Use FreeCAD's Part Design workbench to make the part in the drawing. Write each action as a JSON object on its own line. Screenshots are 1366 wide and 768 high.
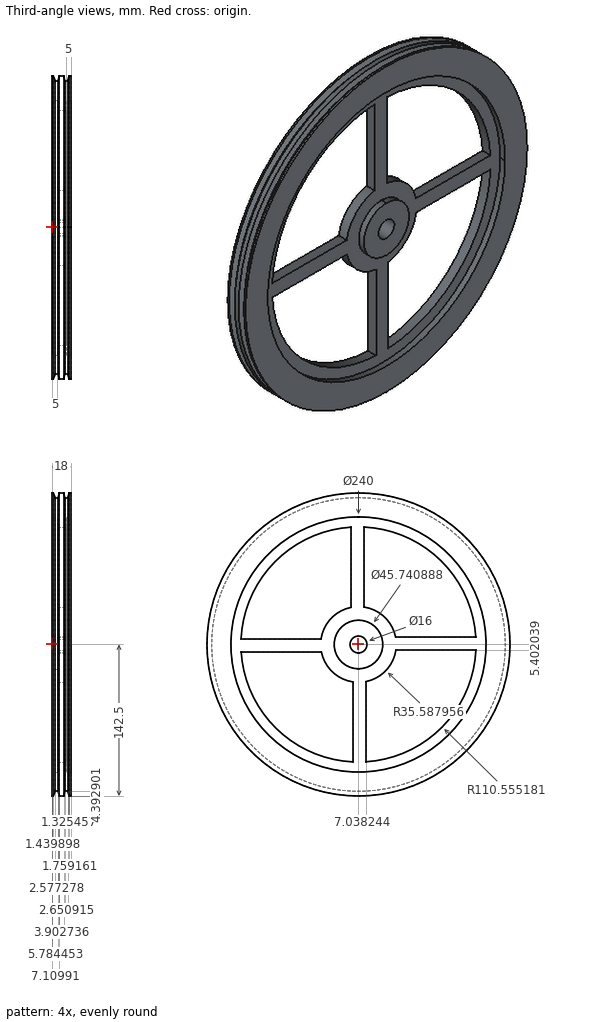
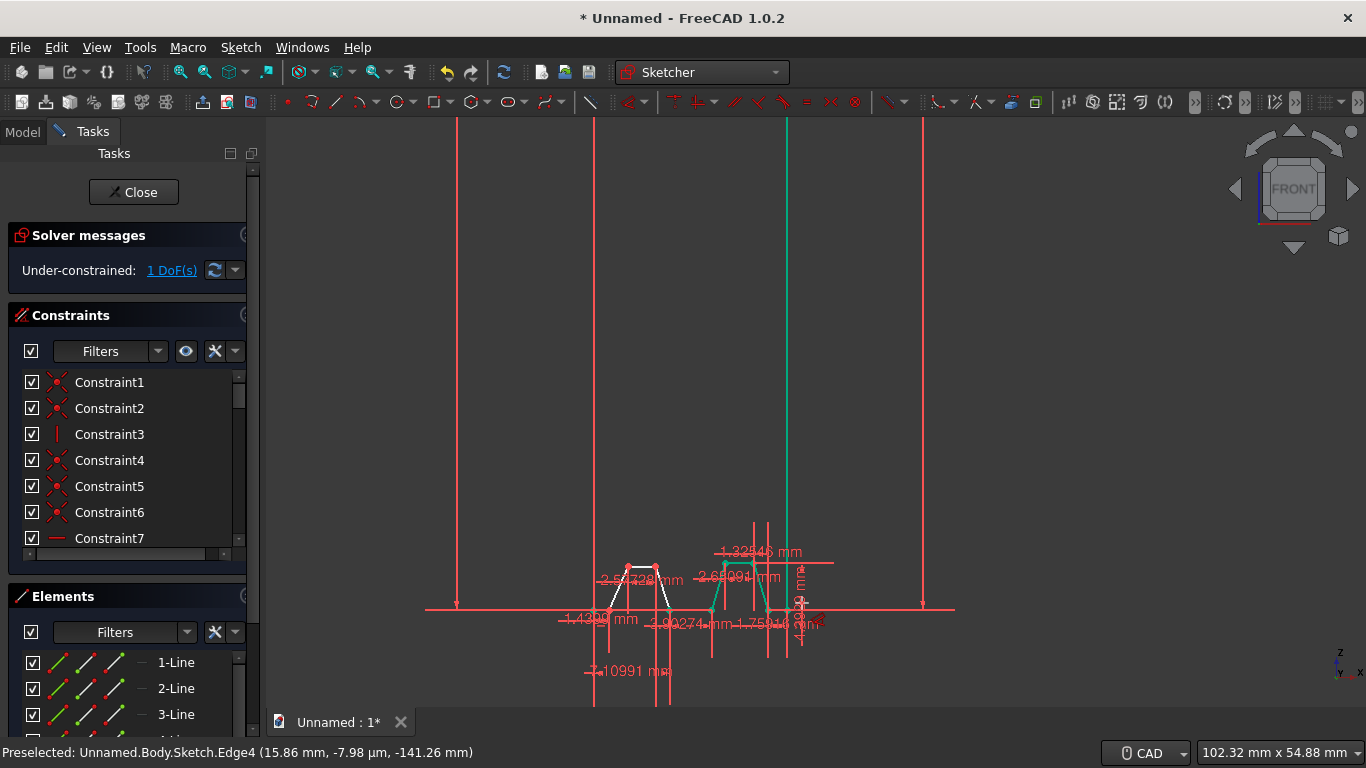
{"action": "left_click", "coordinate": [666, 597]}
{"action": "left_click", "coordinate": [728, 604]}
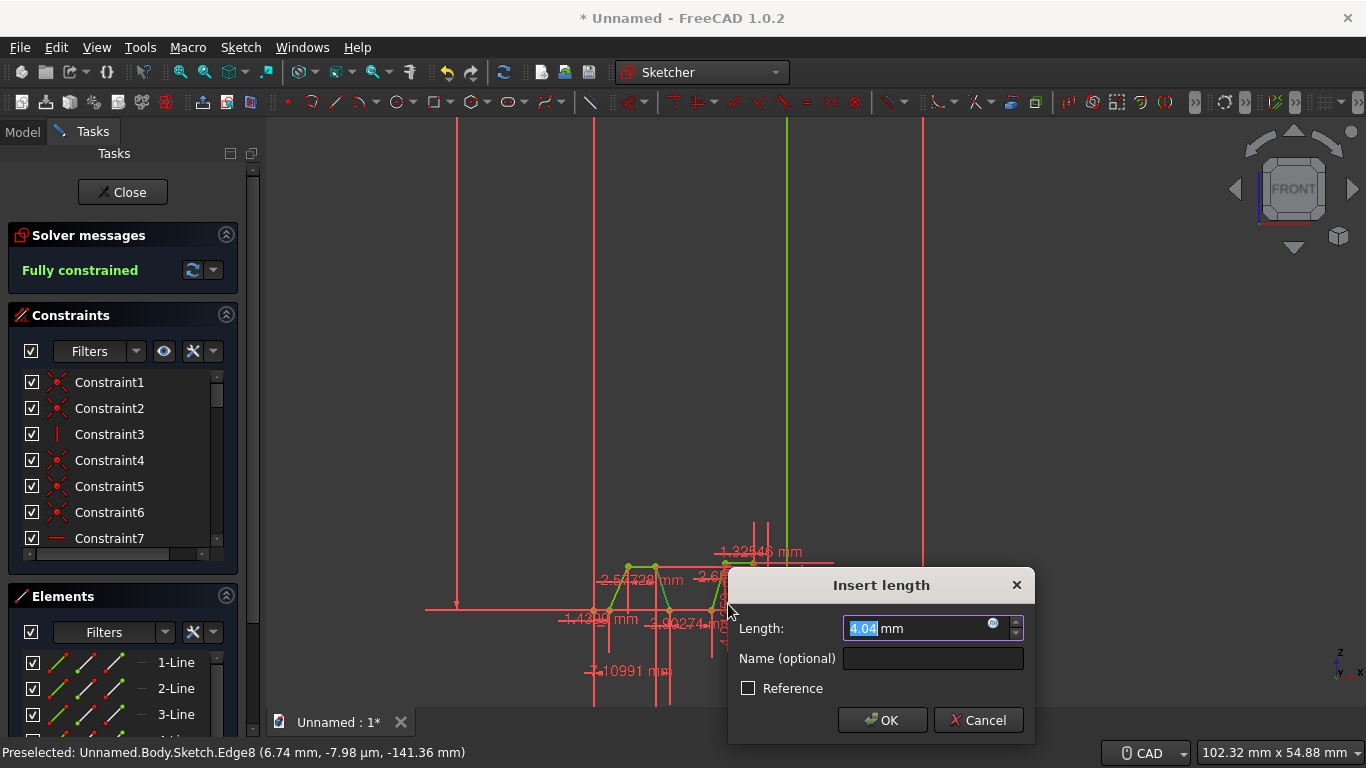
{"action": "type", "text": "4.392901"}
{"action": "key", "text": "Return"}
{"action": "key", "text": "Escape"}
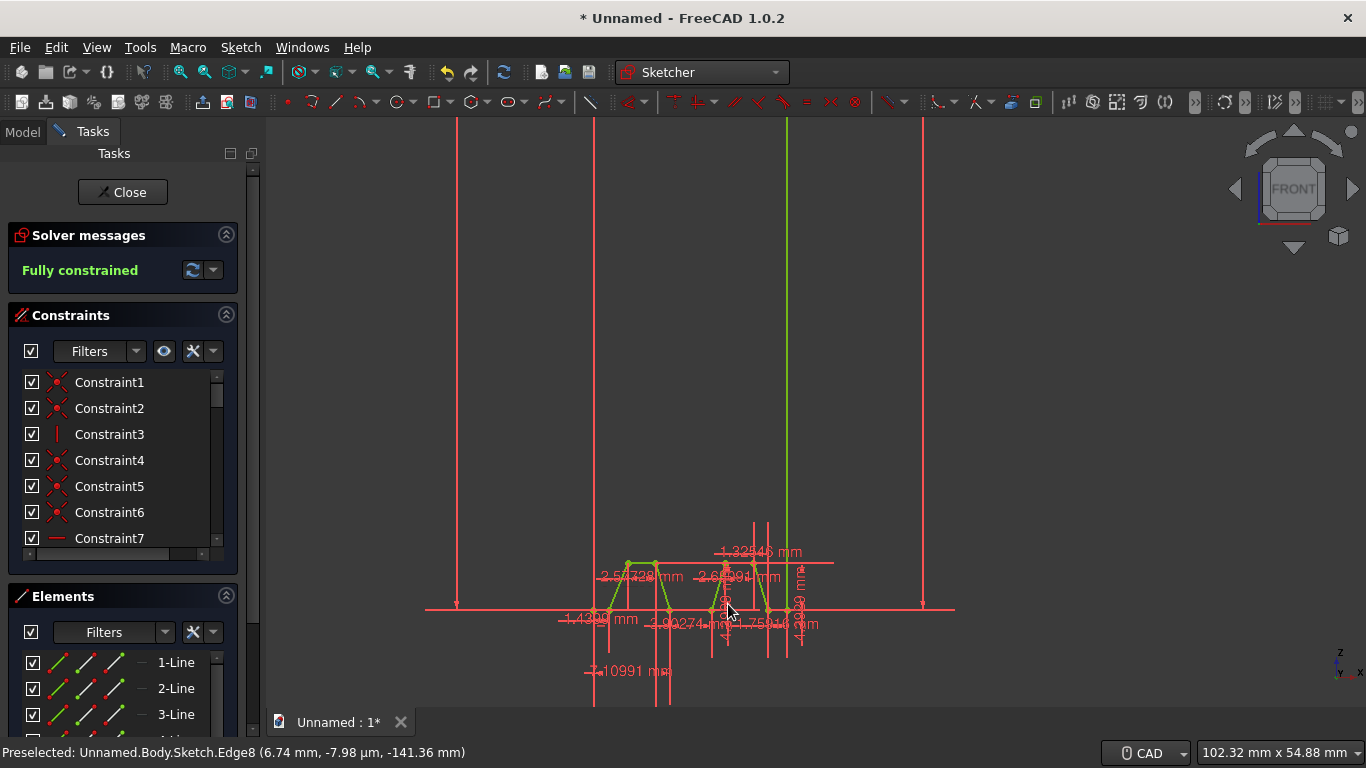
{"action": "left_click", "coordinate": [123, 192]}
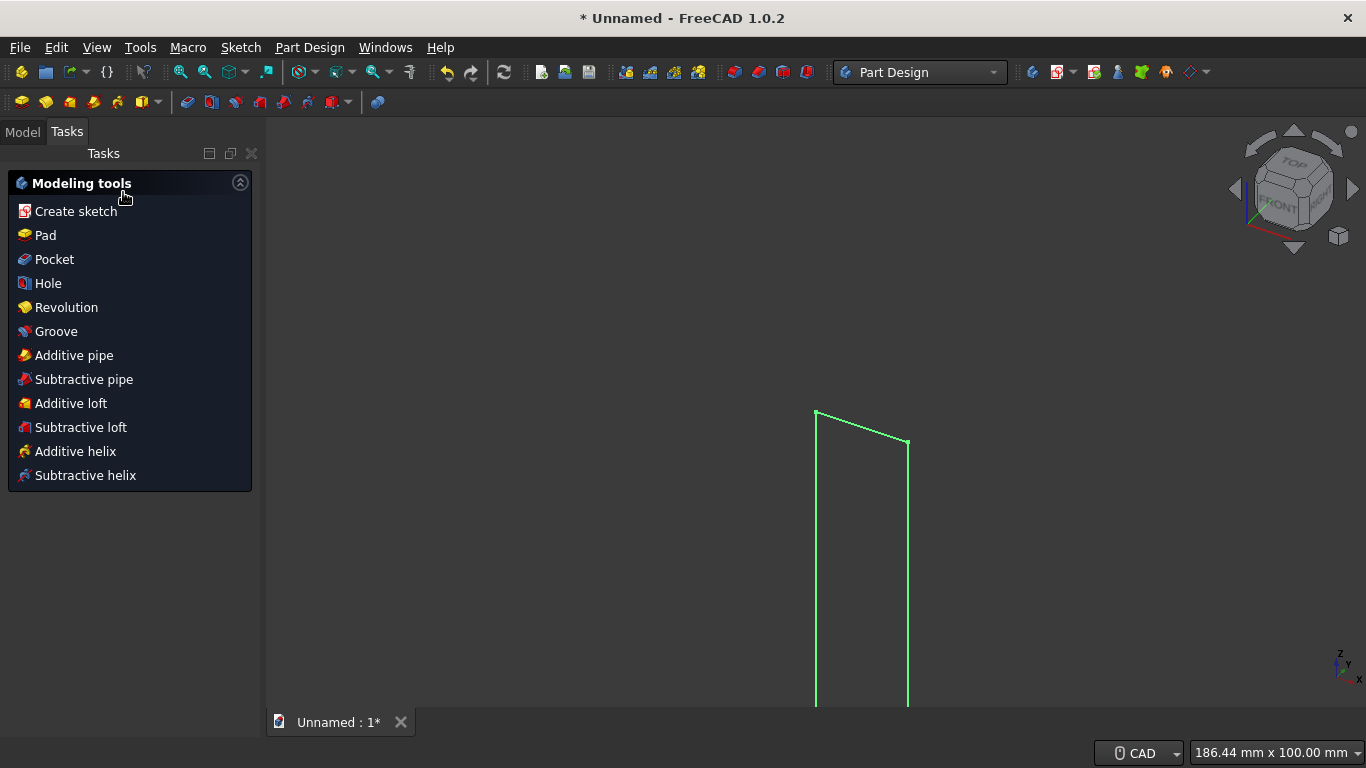
{"action": "left_click", "coordinate": [46, 102]}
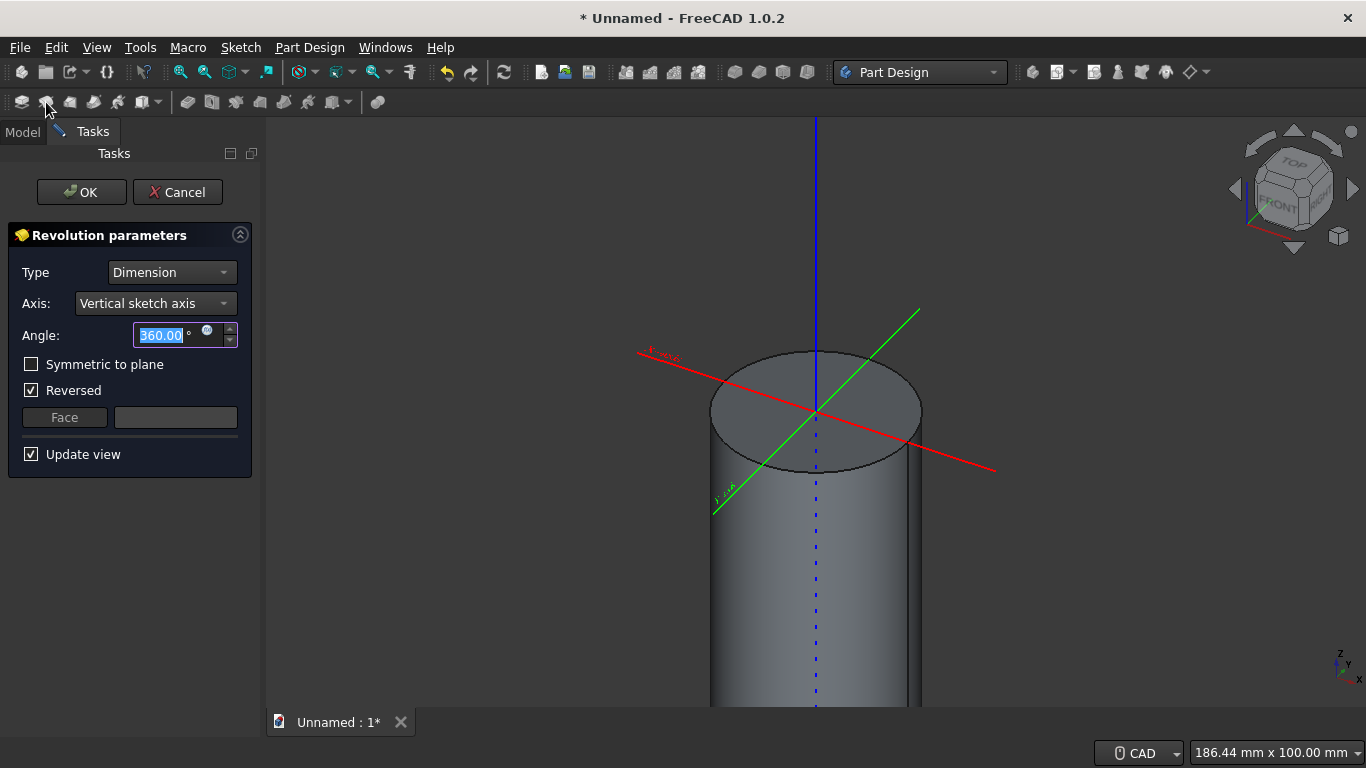
{"action": "left_click", "coordinate": [156, 304]}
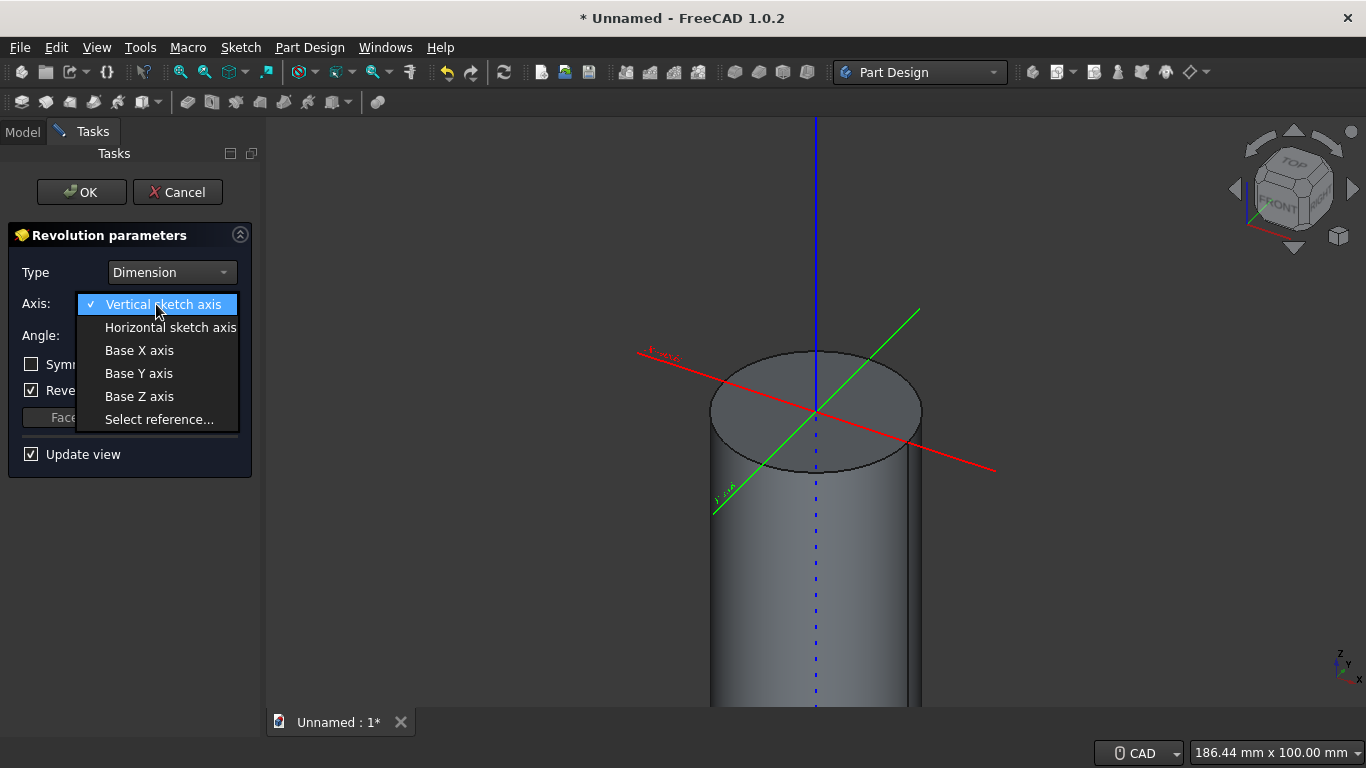
{"action": "left_click", "coordinate": [156, 328]}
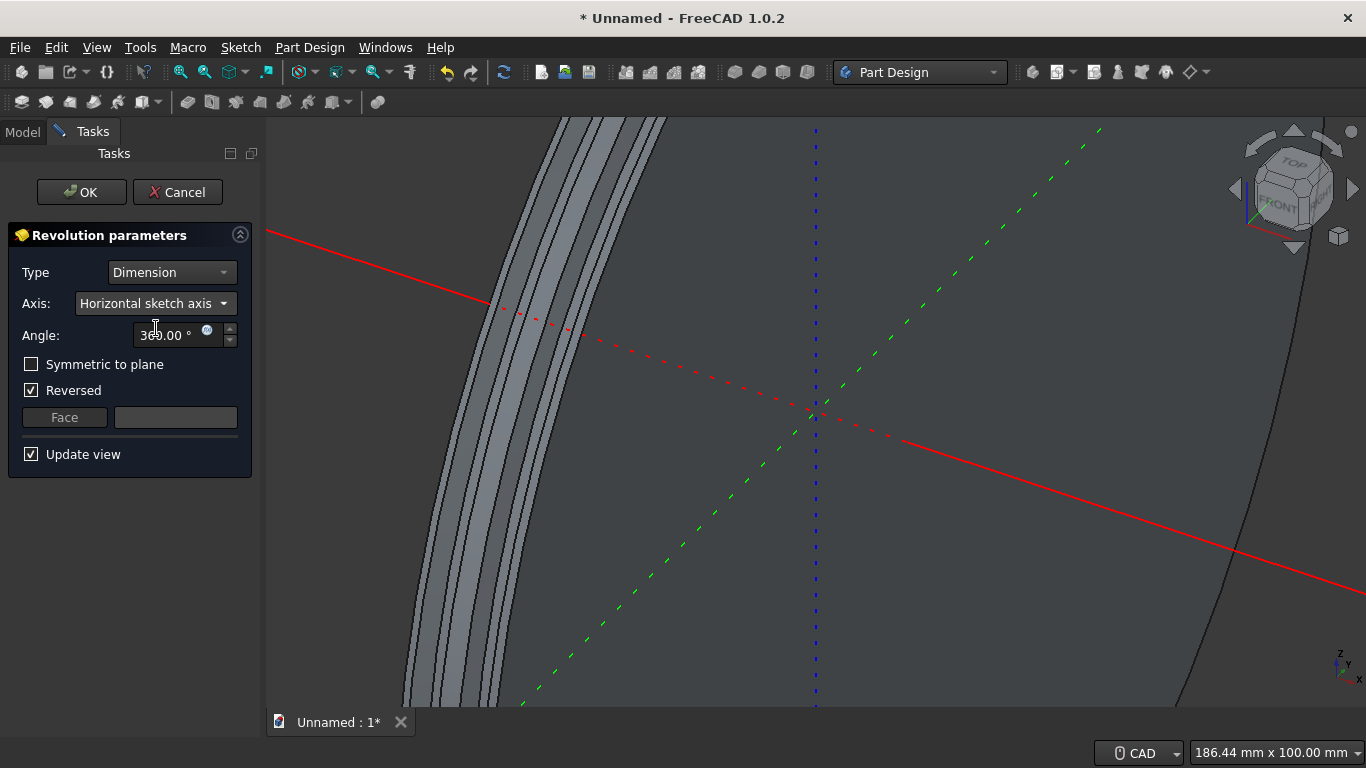
{"action": "left_click", "coordinate": [82, 192]}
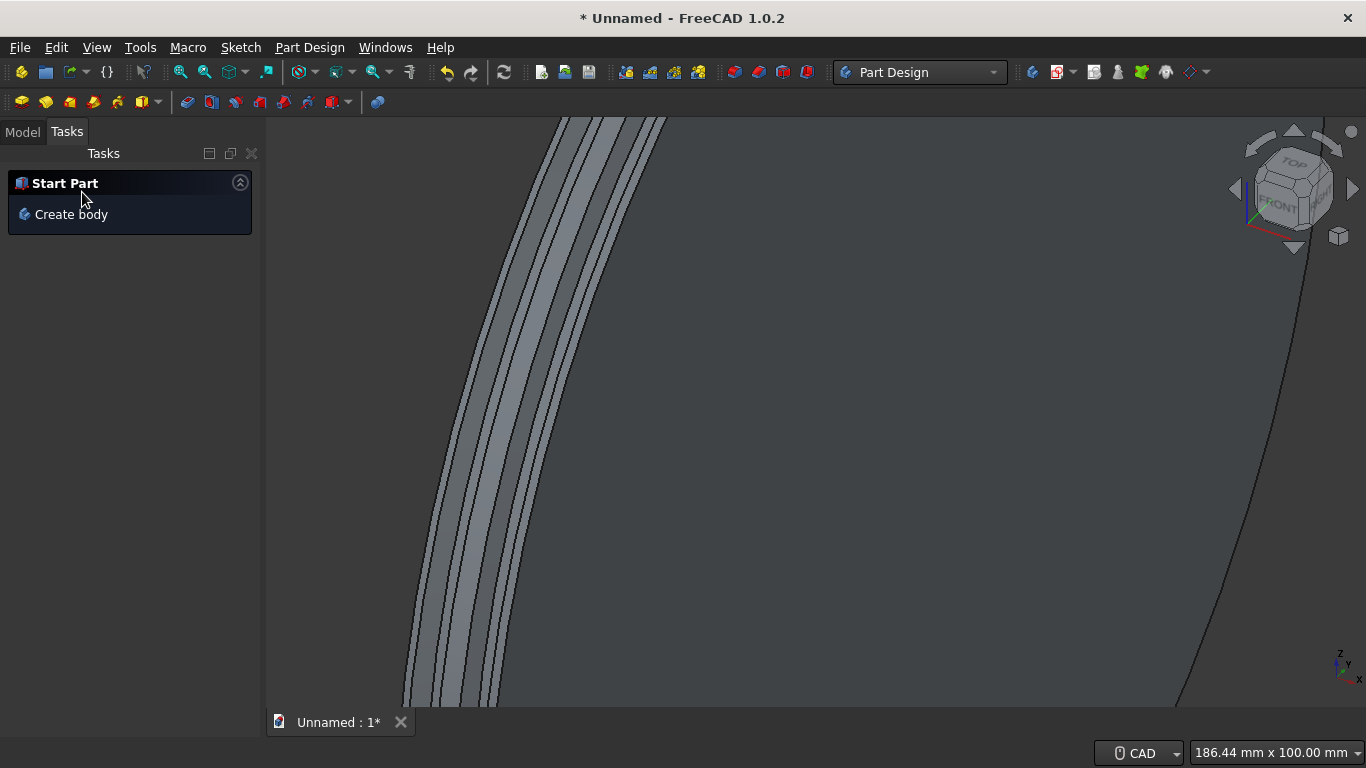
{"action": "left_click", "coordinate": [182, 72]}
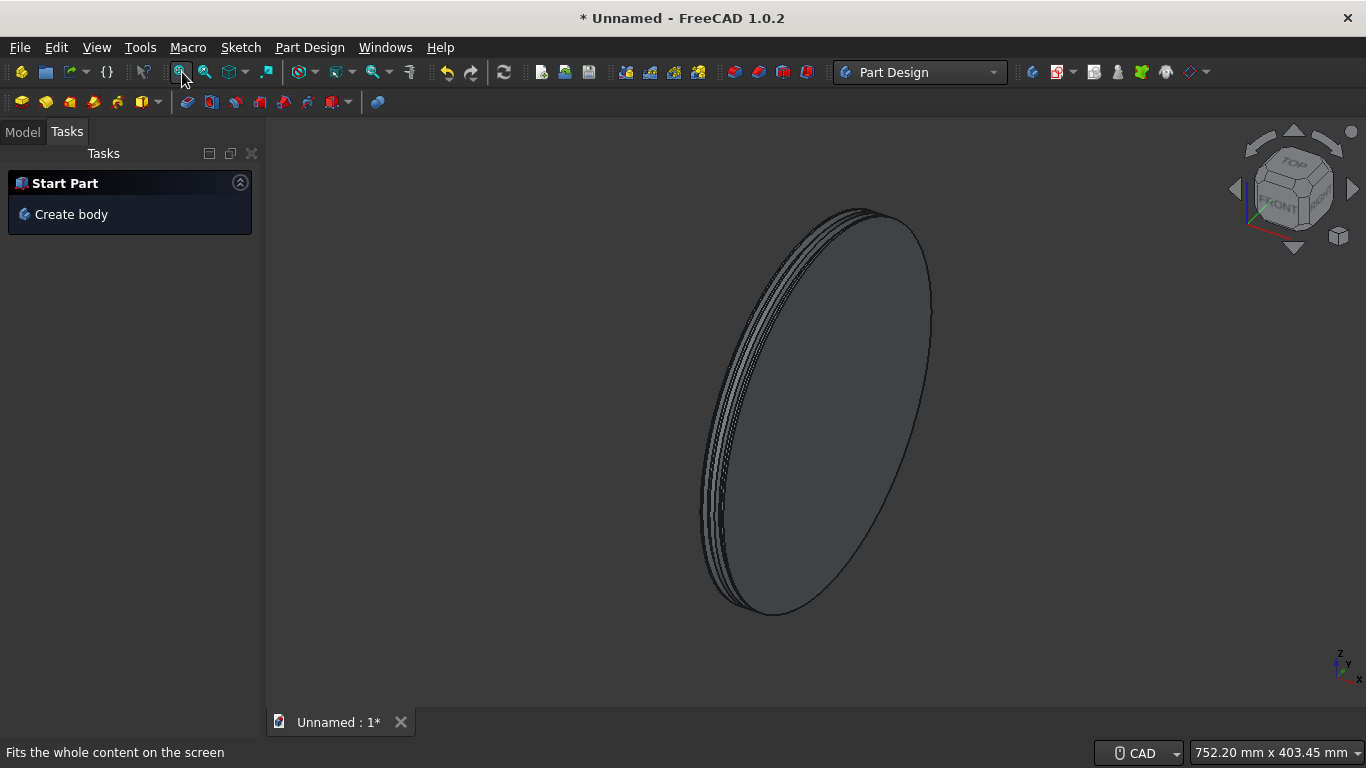
{"action": "key", "text": "6"}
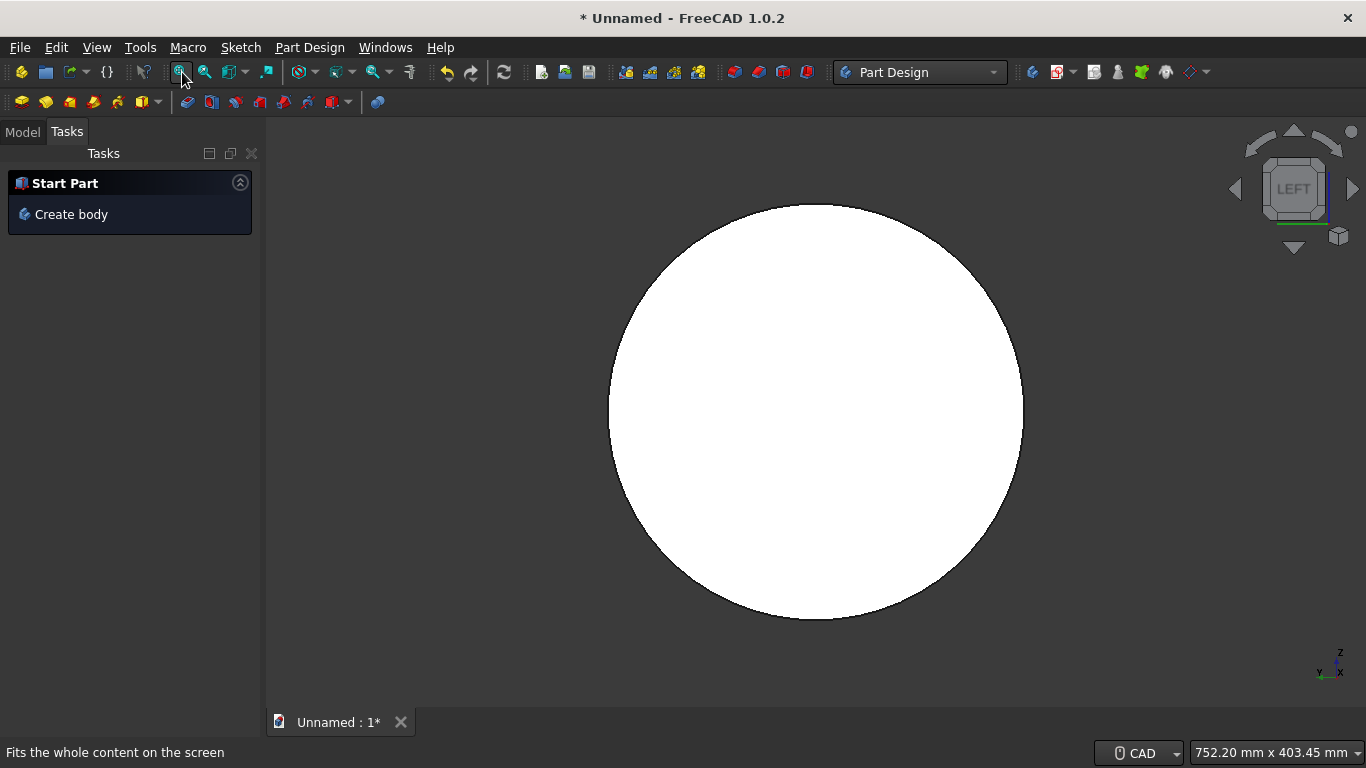
{"action": "left_click", "coordinate": [816, 411]}